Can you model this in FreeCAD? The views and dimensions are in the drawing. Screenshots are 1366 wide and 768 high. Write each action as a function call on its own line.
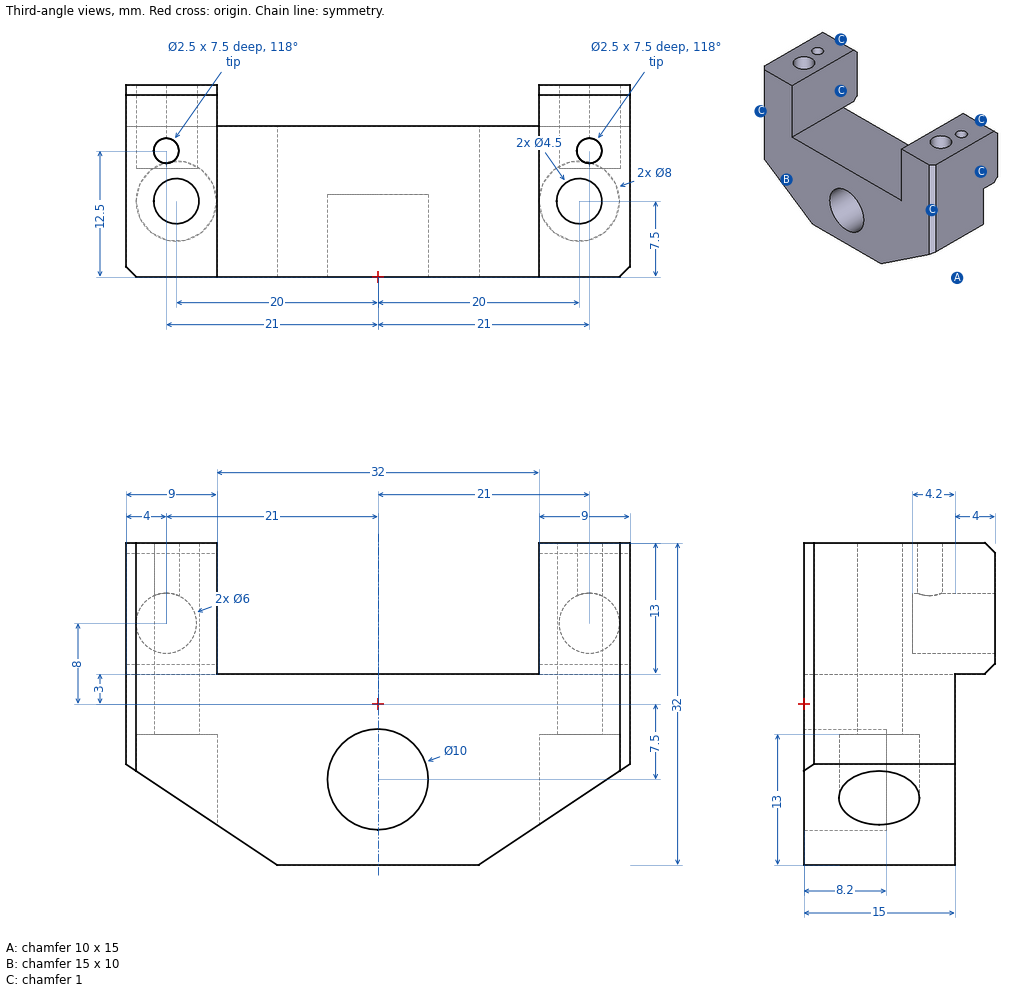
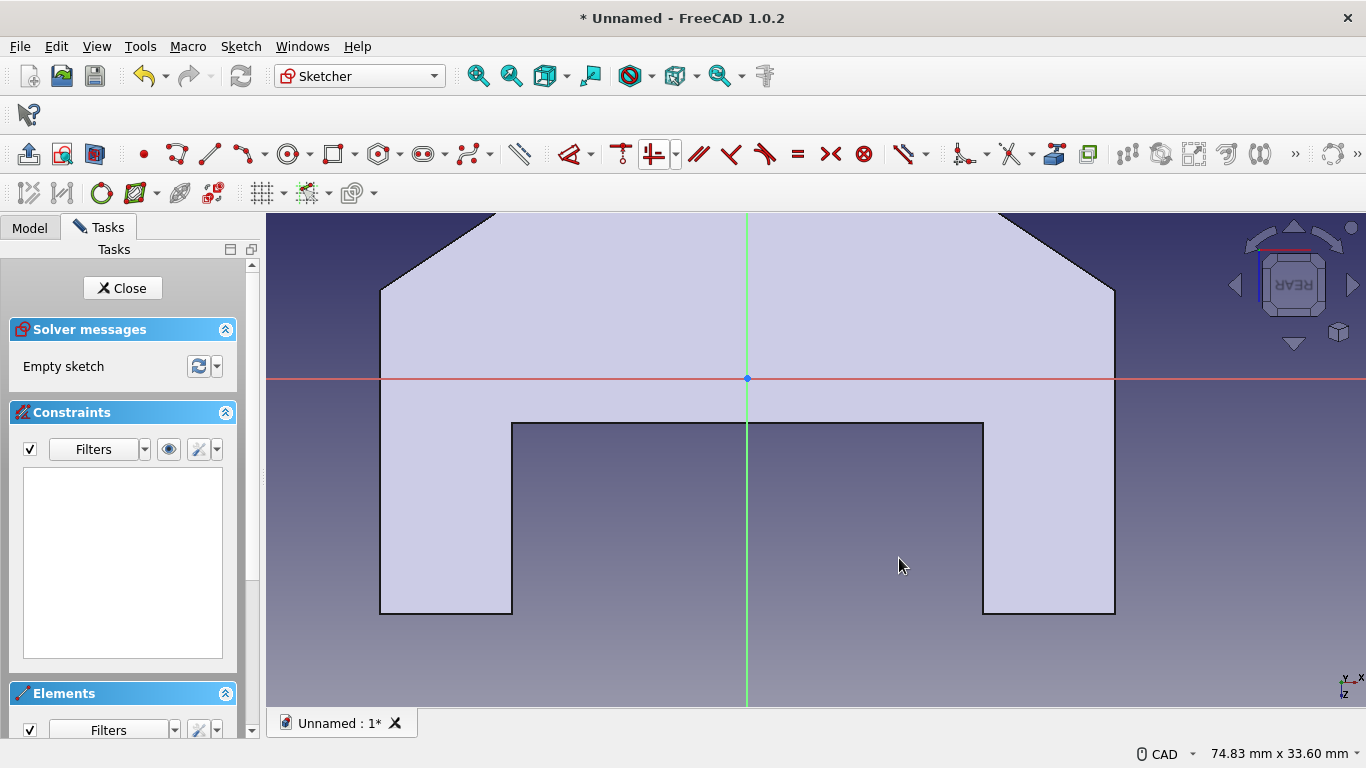
click(288, 154)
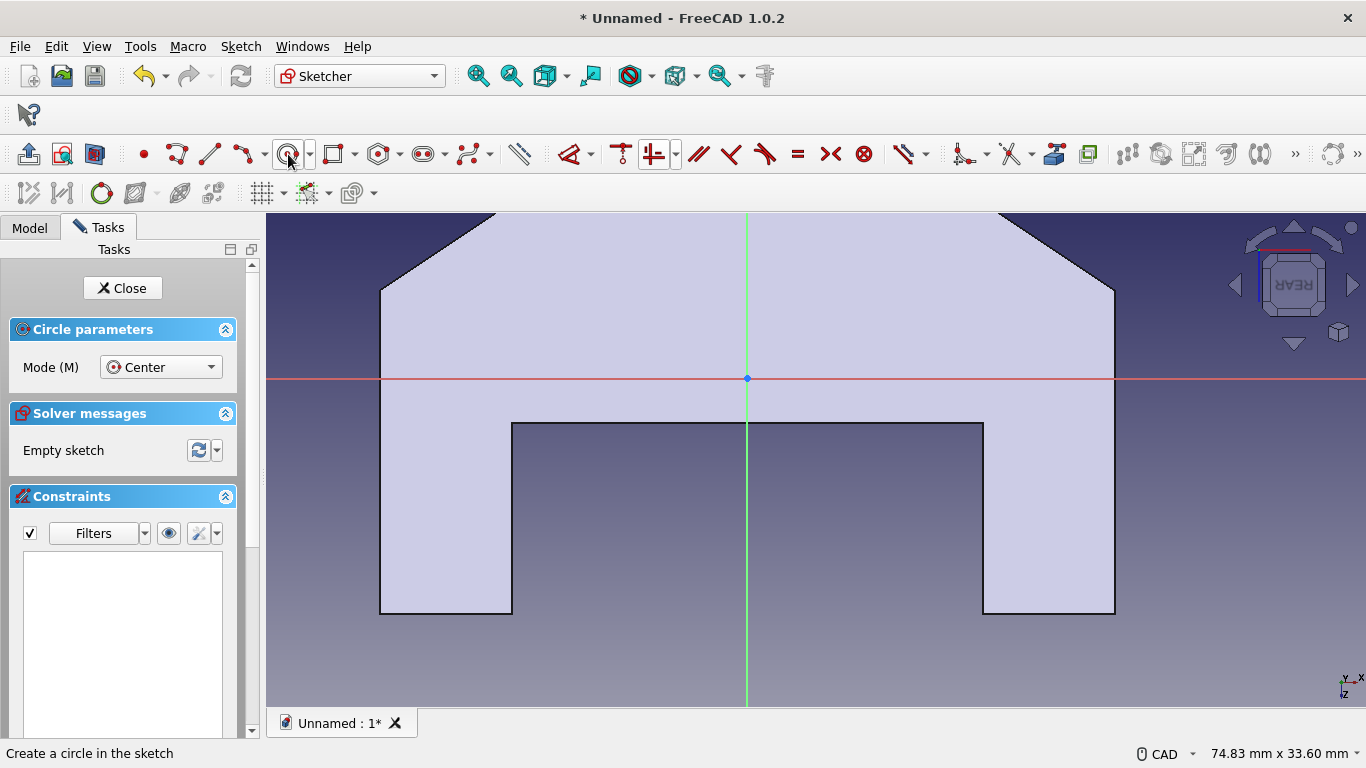
click(439, 496)
move(470, 465)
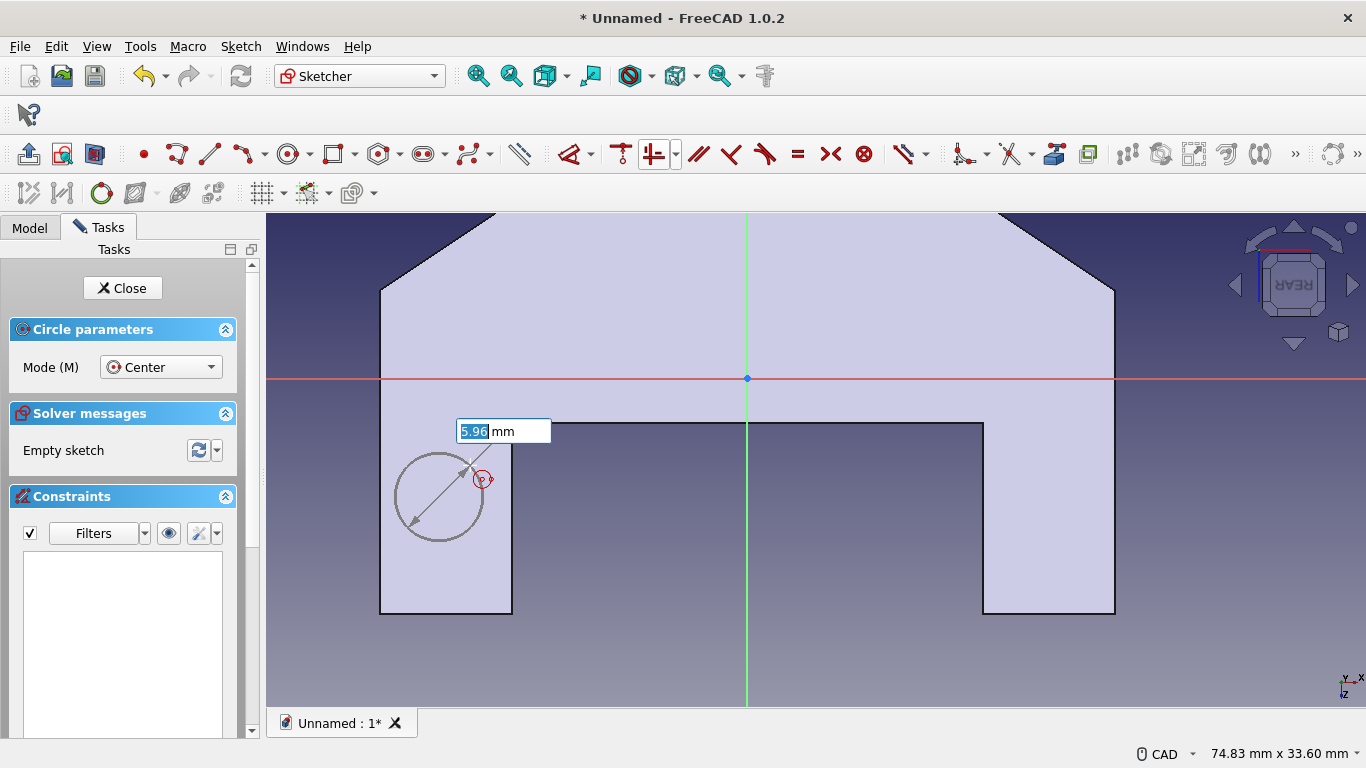
text(6)
key(Return)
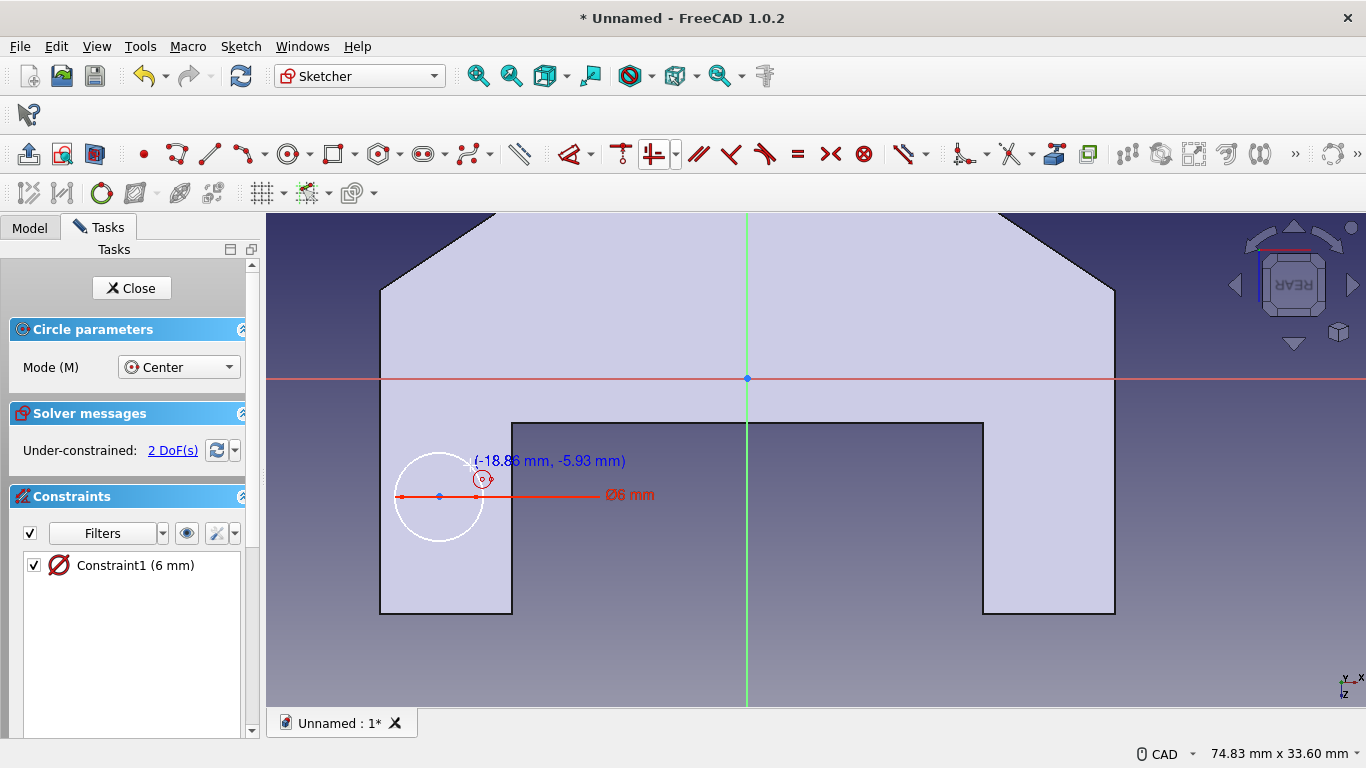
click(1056, 496)
move(1087, 465)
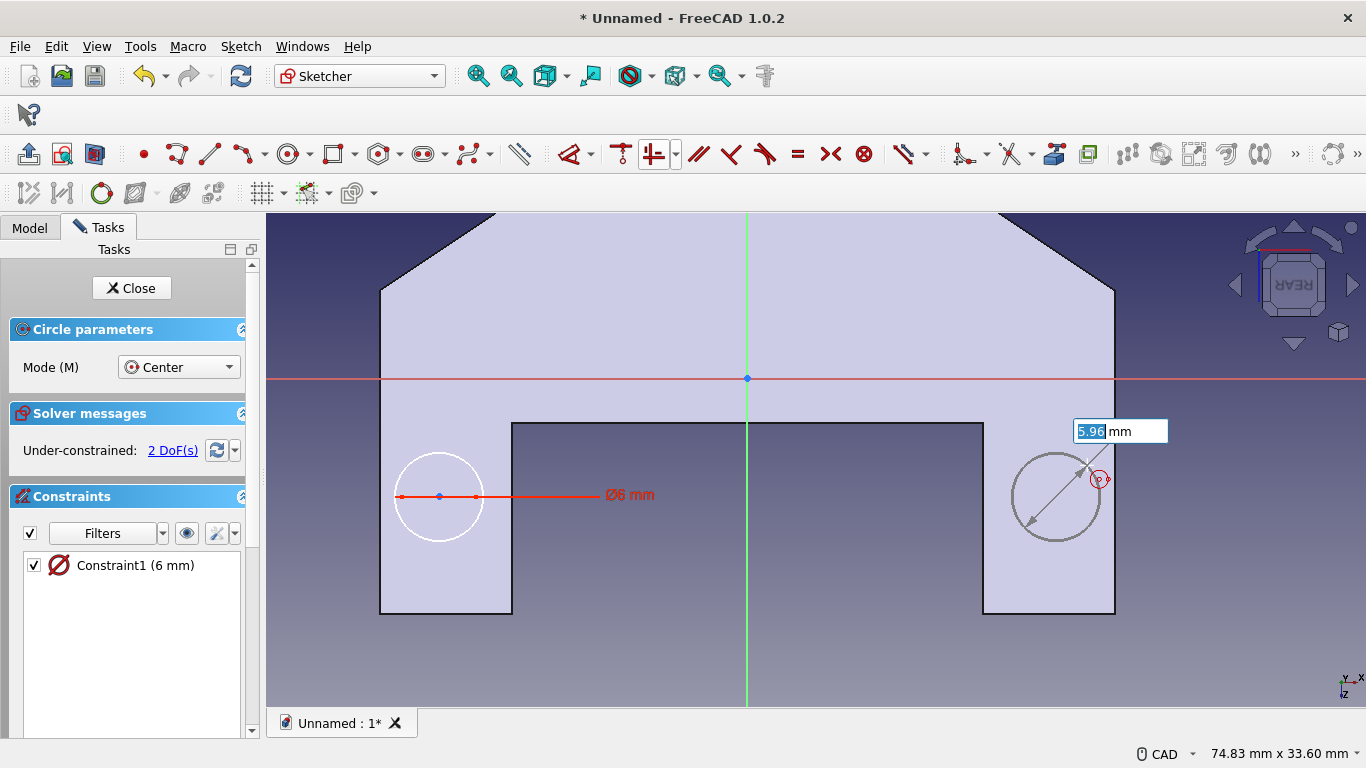
text(6)
key(Return)
key(Escape)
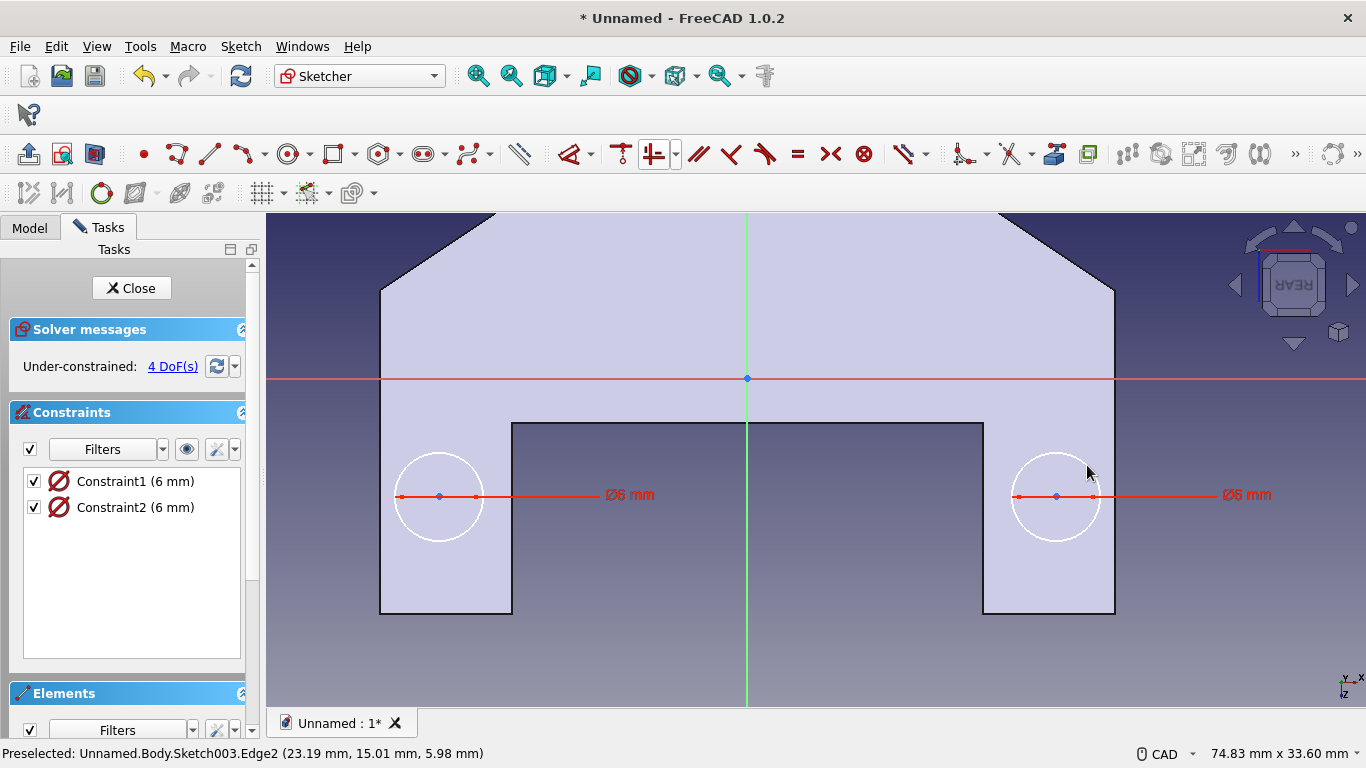
click(439, 497)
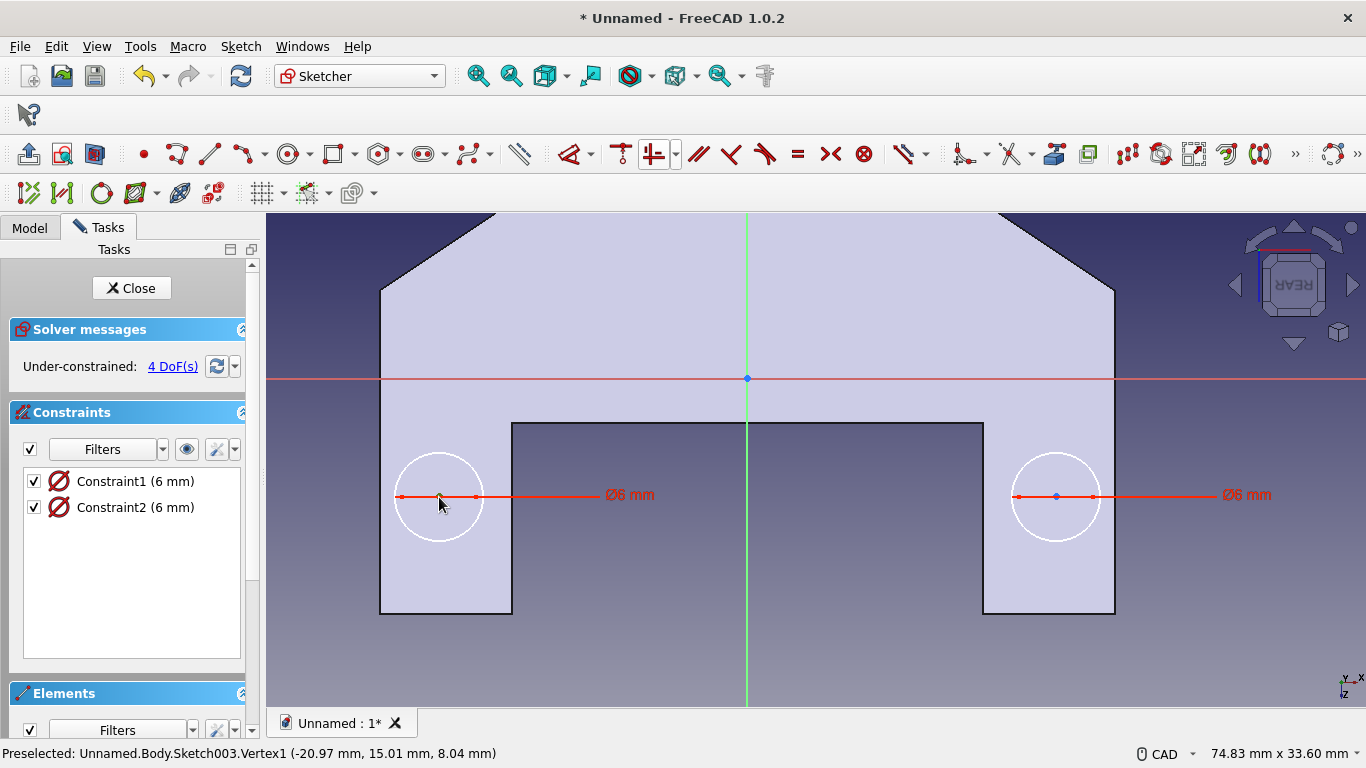
click(1056, 497)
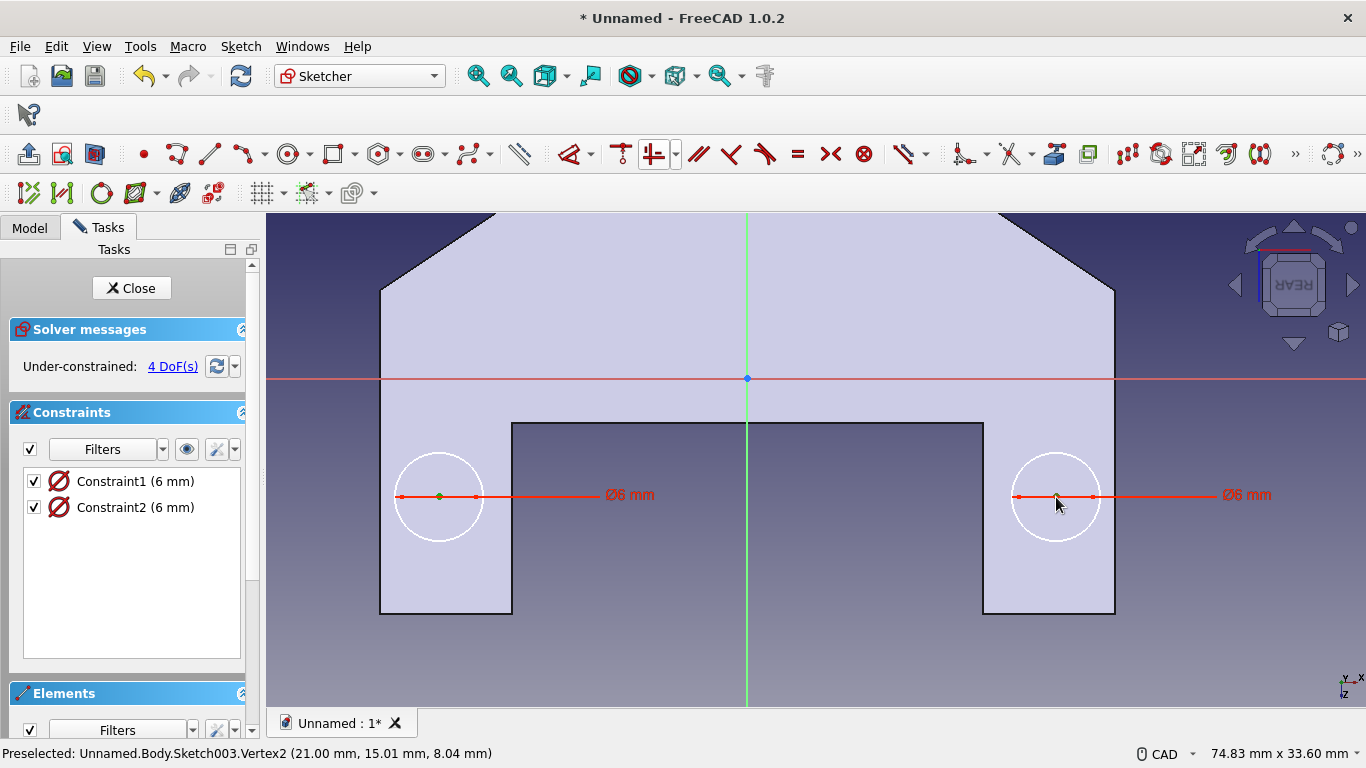
key(h)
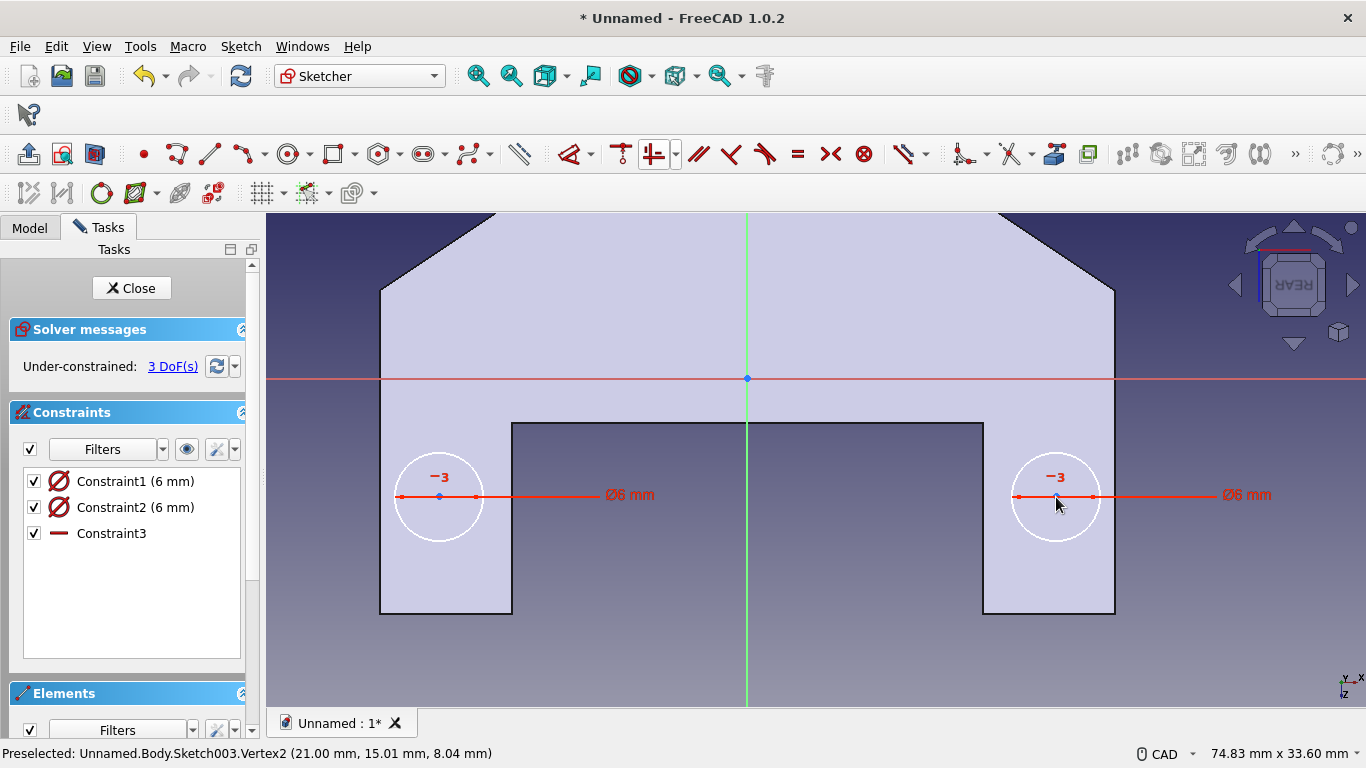
click(568, 154)